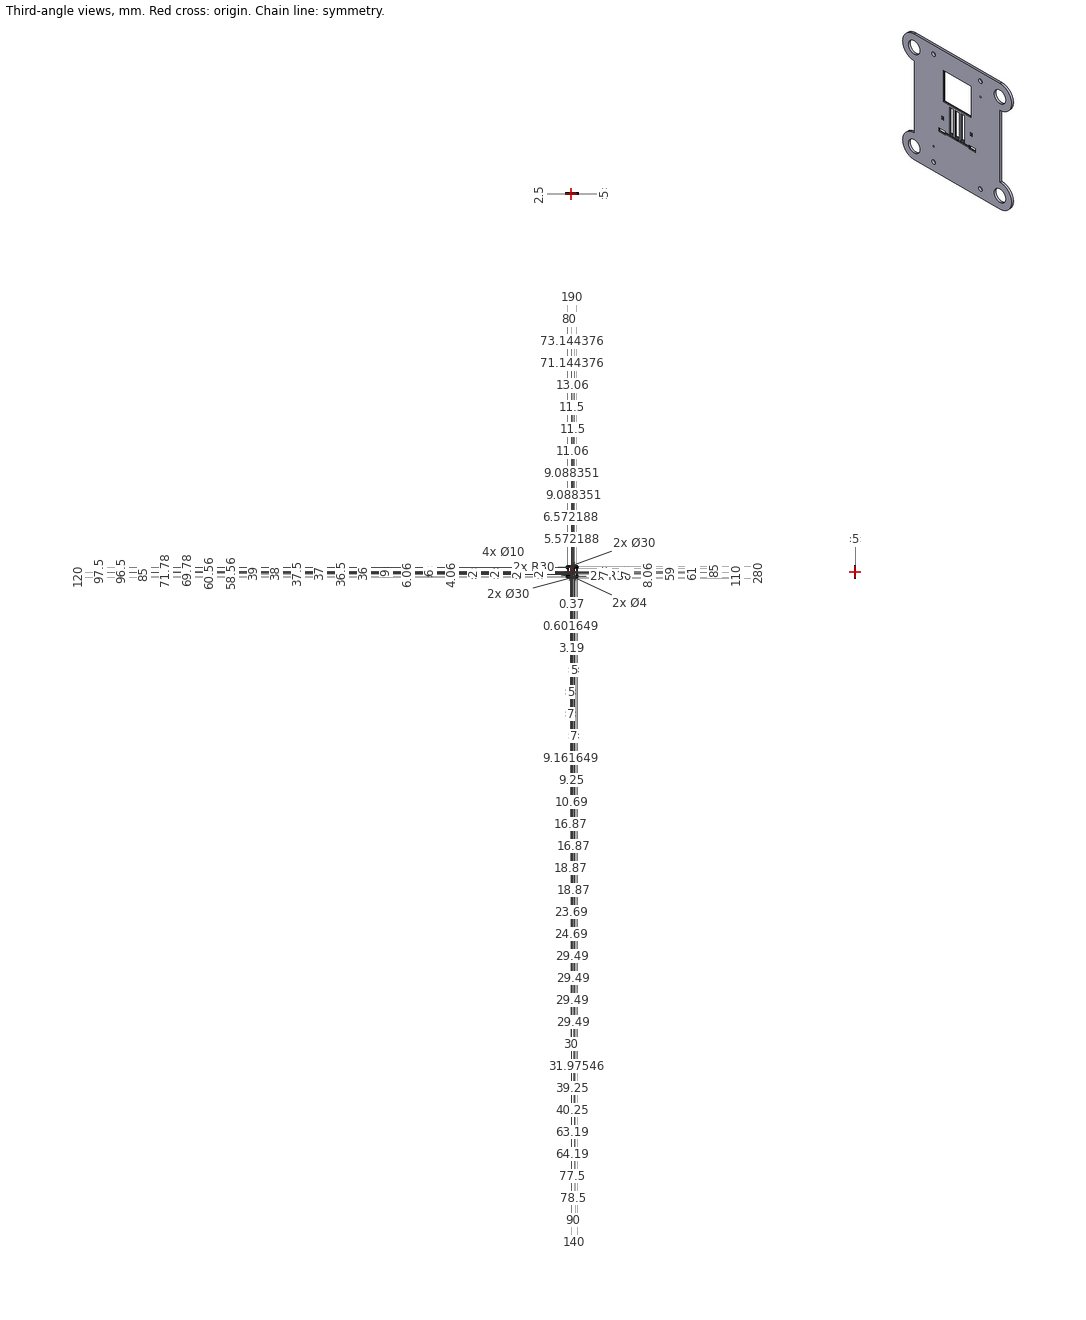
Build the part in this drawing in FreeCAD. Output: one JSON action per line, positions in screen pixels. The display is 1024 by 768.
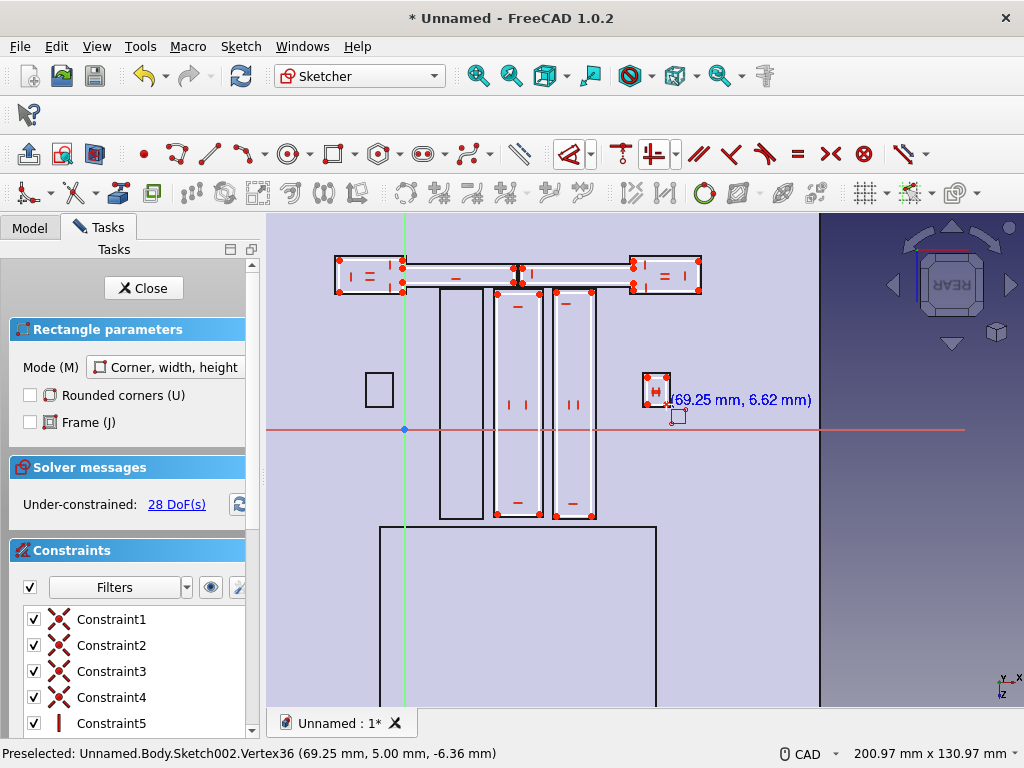
{"action": "left_click", "coordinate": [384, 531]}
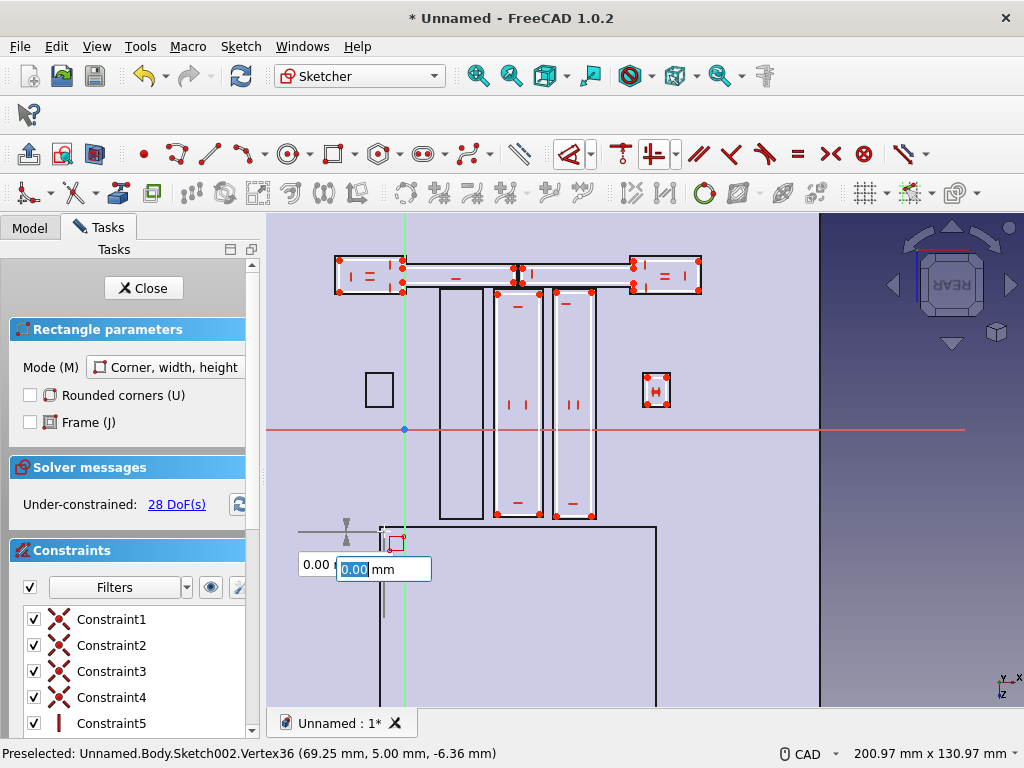
{"action": "scroll", "coordinate": [648, 379], "scroll_direction": "down", "scroll_amount": 3}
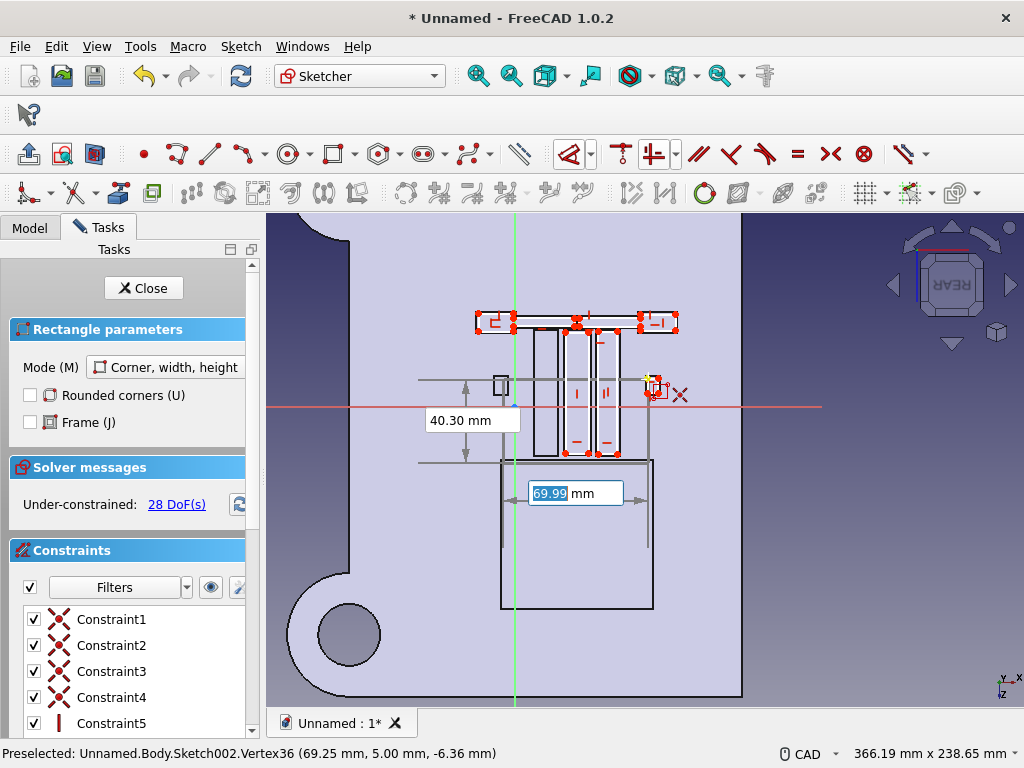
{"action": "left_click", "coordinate": [651, 607]}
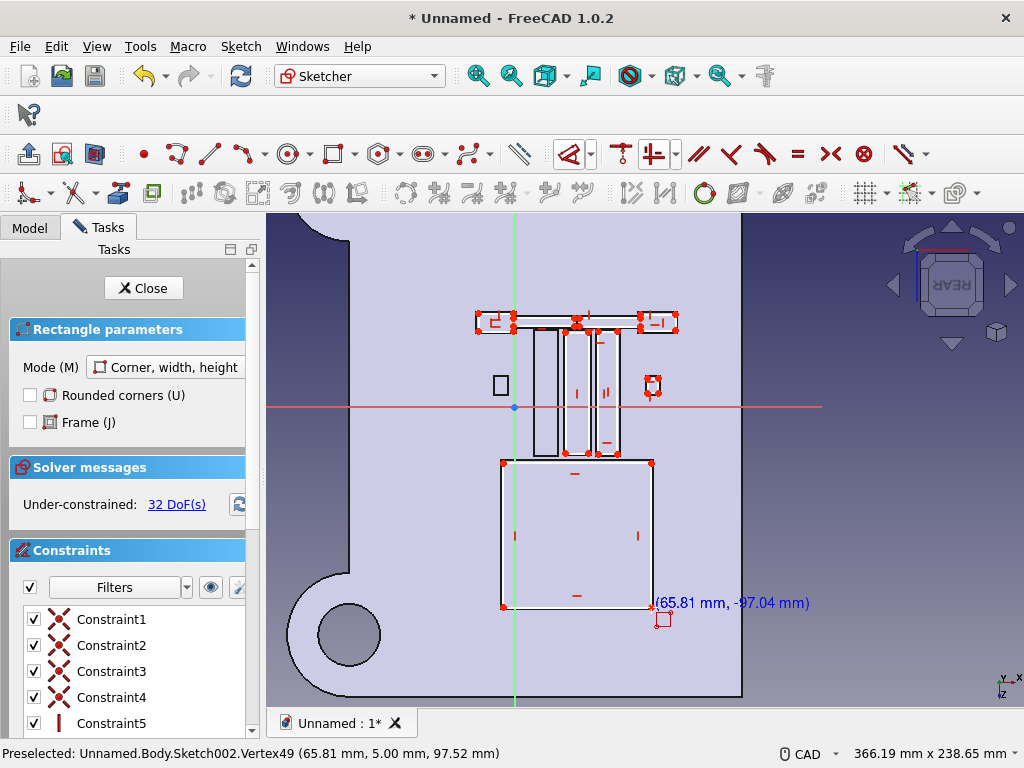
{"action": "scroll", "coordinate": [537, 332], "scroll_direction": "up", "scroll_amount": 6}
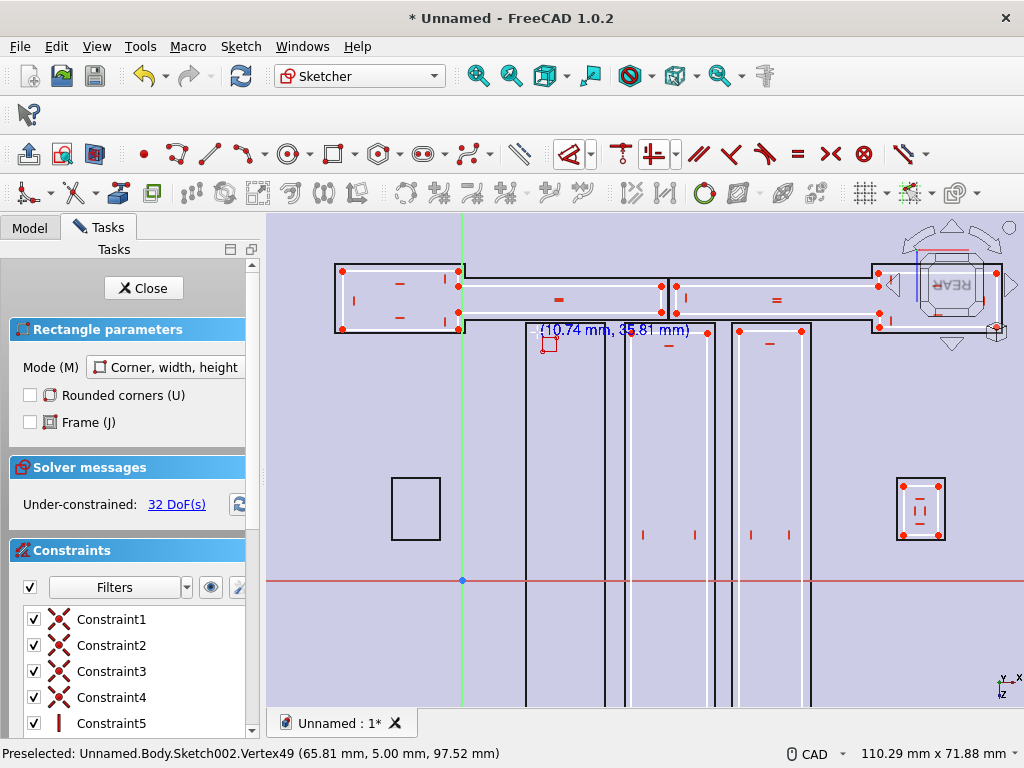
{"action": "left_click", "coordinate": [536, 330]}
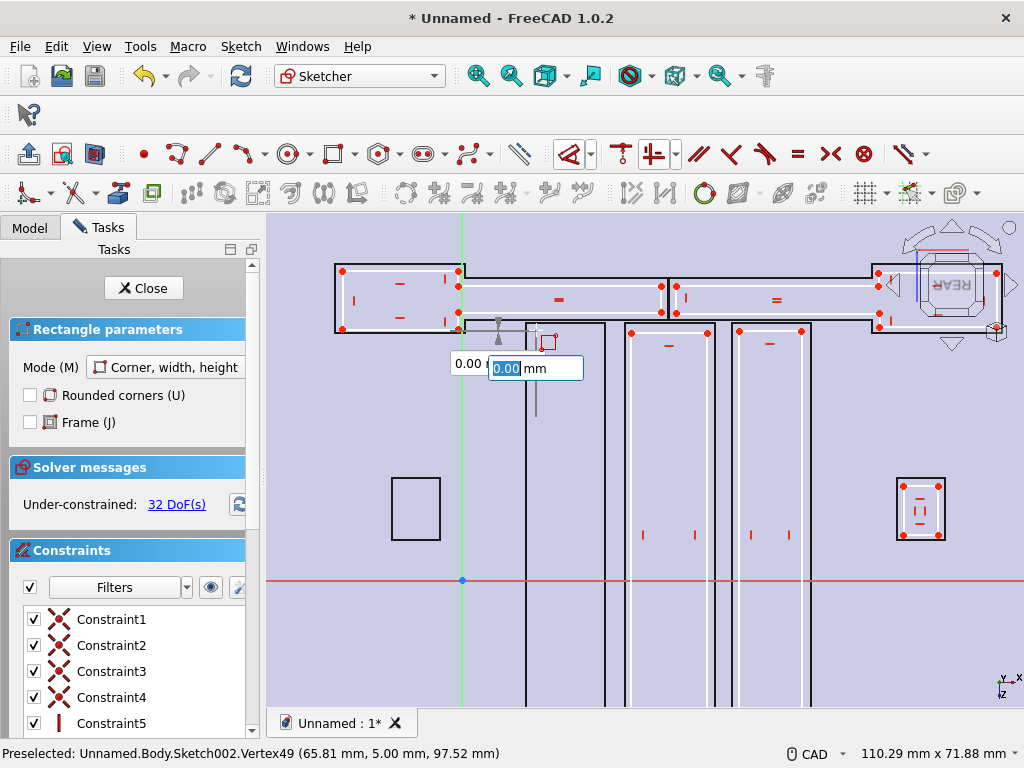
{"action": "scroll", "coordinate": [537, 332], "scroll_direction": "down", "scroll_amount": 6}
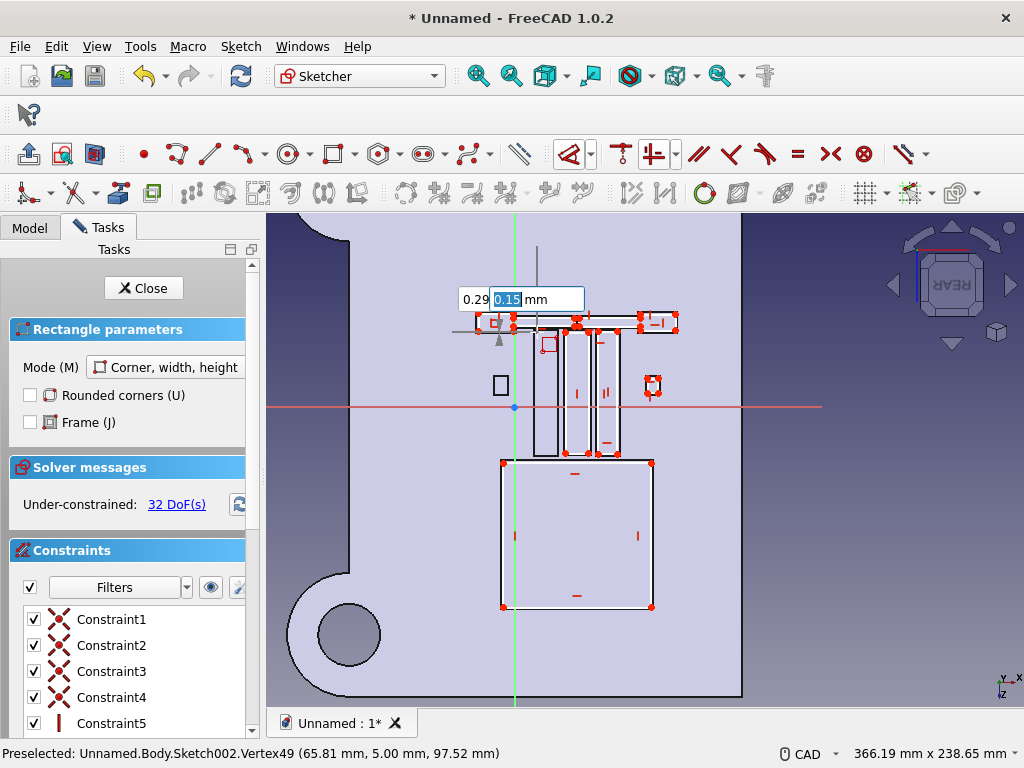
{"action": "scroll", "coordinate": [556, 454], "scroll_direction": "up", "scroll_amount": 3}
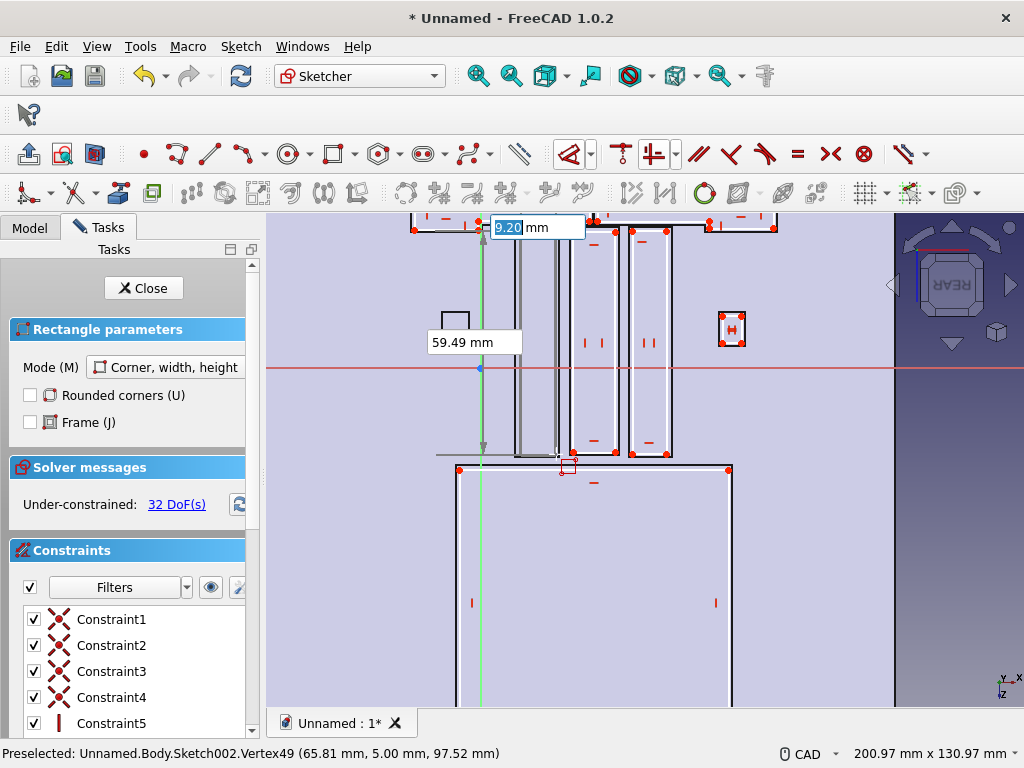
{"action": "left_click", "coordinate": [555, 453]}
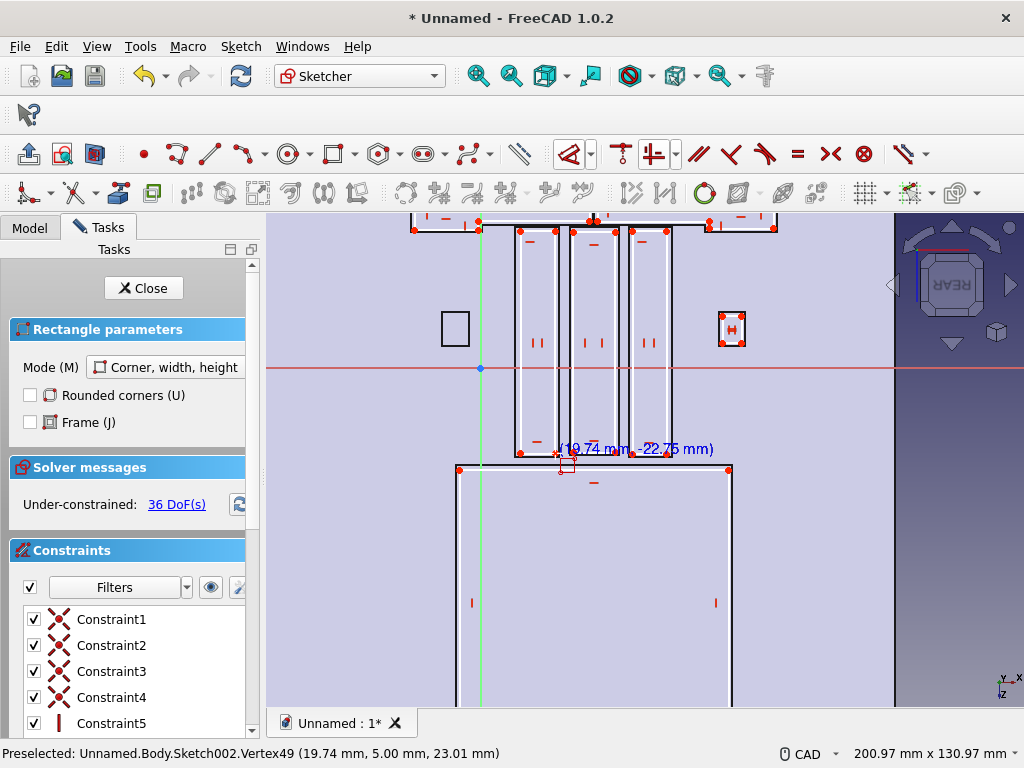
{"action": "left_click", "coordinate": [446, 315]}
{"action": "left_click", "coordinate": [465, 342]}
{"action": "key", "text": "Escape"}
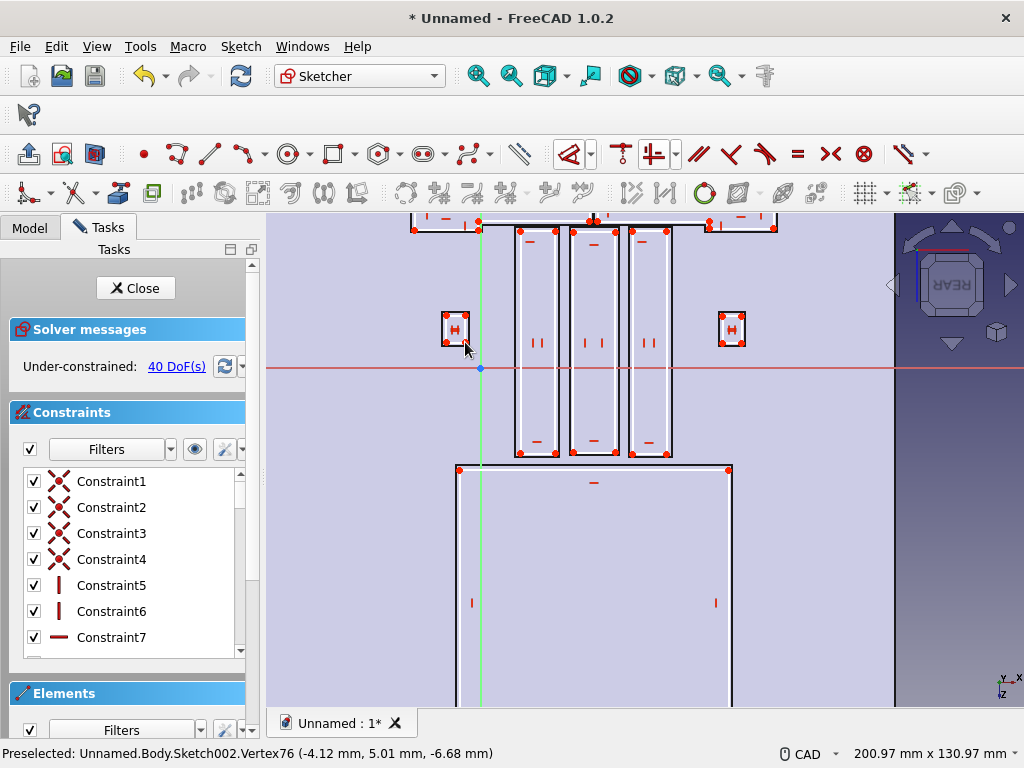
{"action": "scroll", "coordinate": [556, 454], "scroll_direction": "down", "scroll_amount": 3}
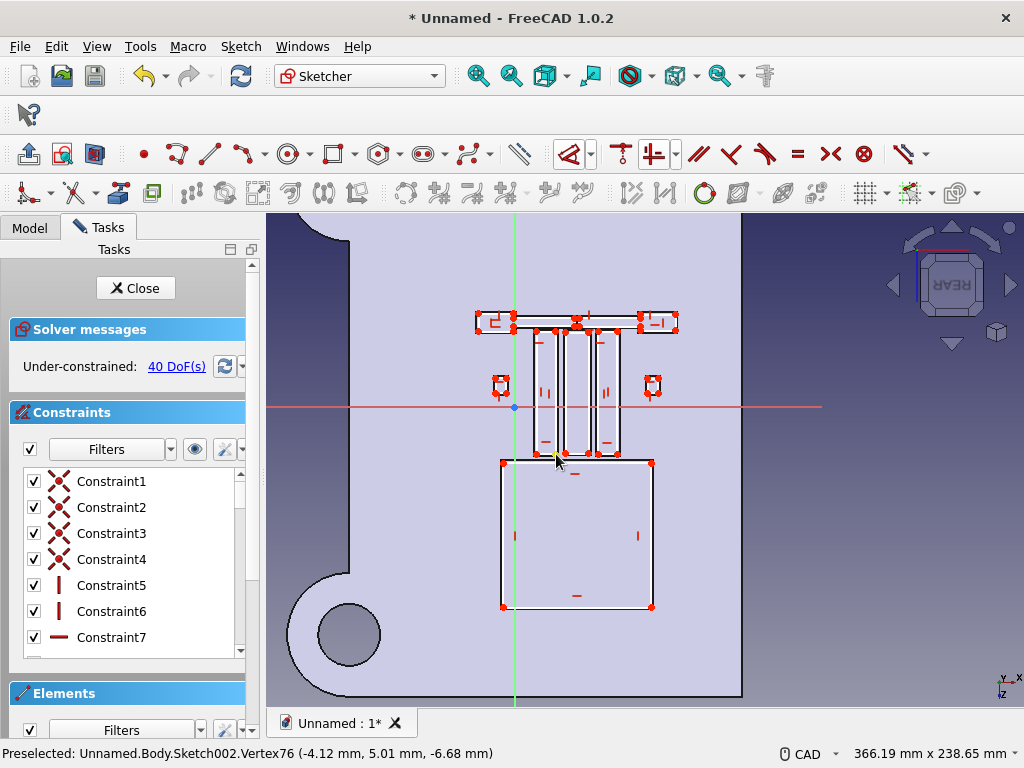
{"action": "scroll", "coordinate": [514, 329], "scroll_direction": "up", "scroll_amount": 12}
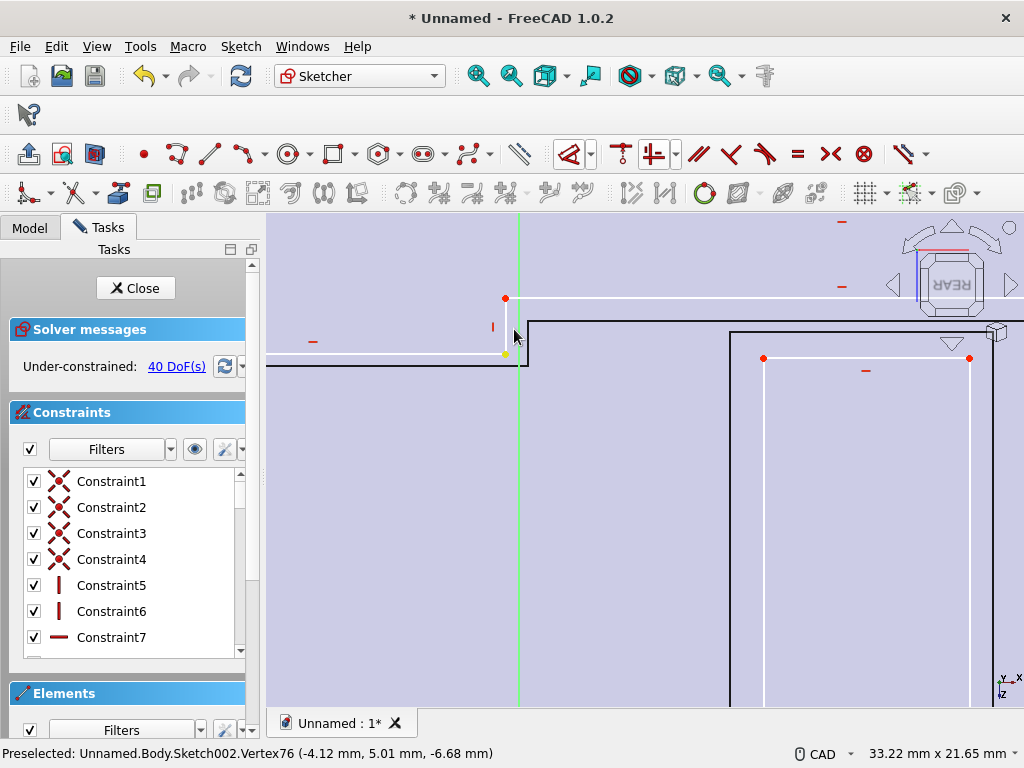
{"action": "left_click", "coordinate": [506, 326]}